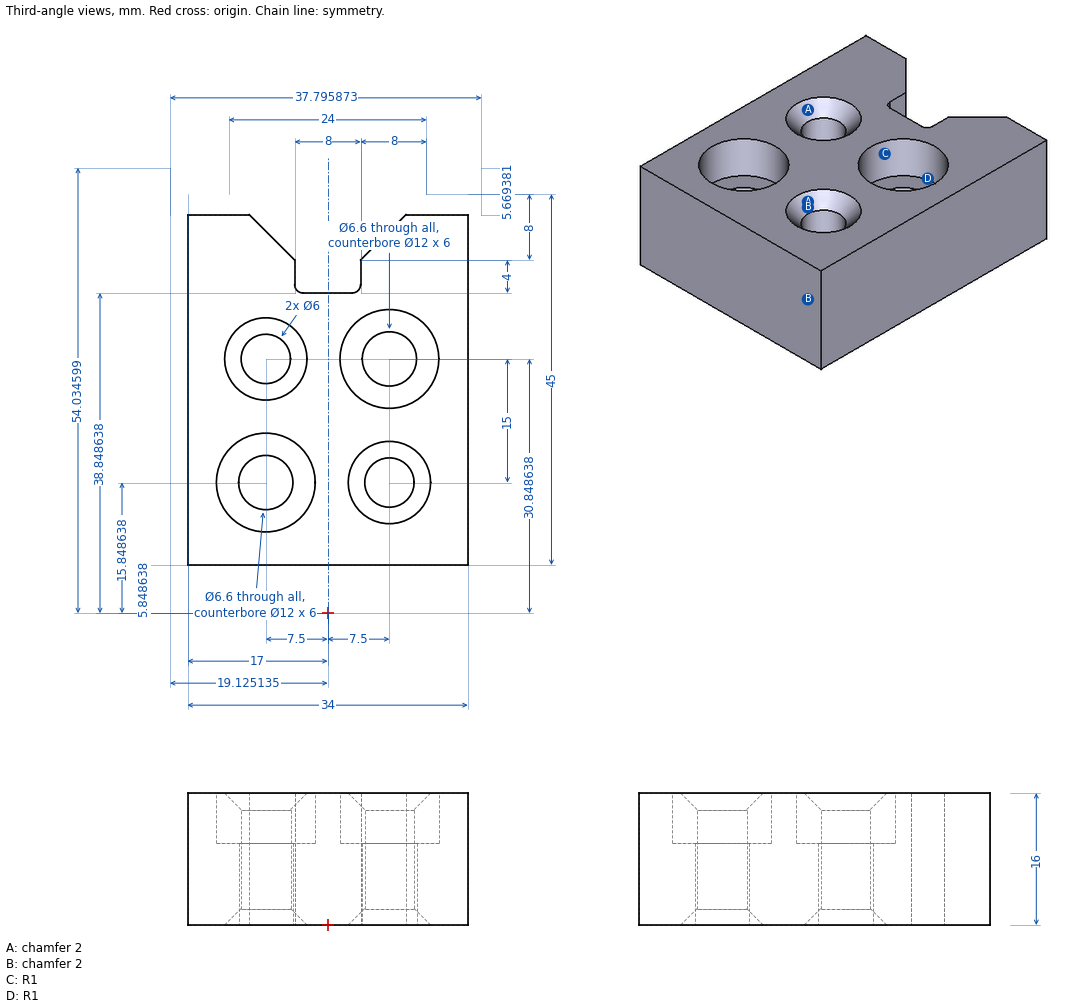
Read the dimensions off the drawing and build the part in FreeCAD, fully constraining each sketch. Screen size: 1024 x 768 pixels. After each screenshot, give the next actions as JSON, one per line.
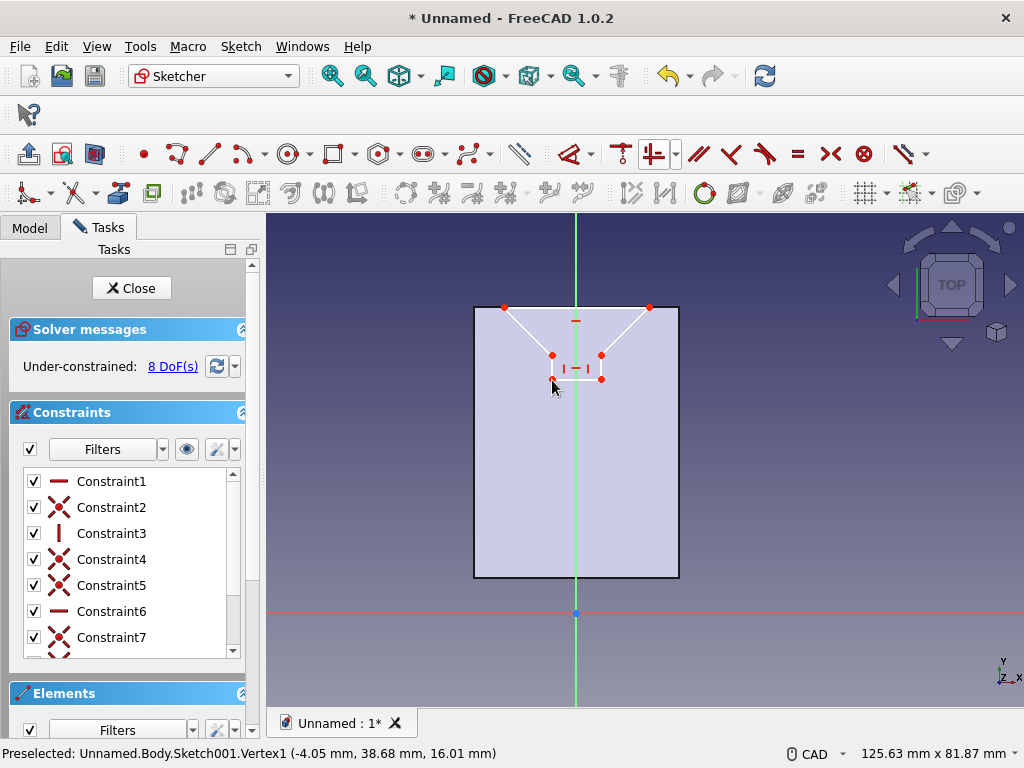
{"action": "left_click", "coordinate": [601, 356]}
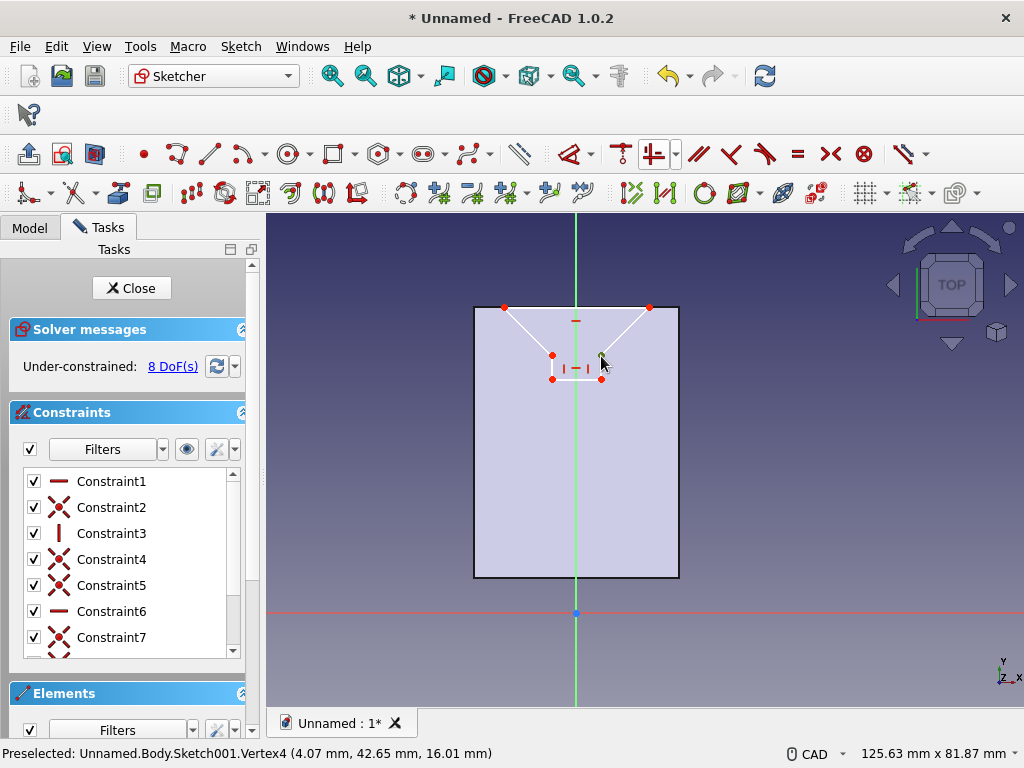
{"action": "left_click", "coordinate": [552, 356]}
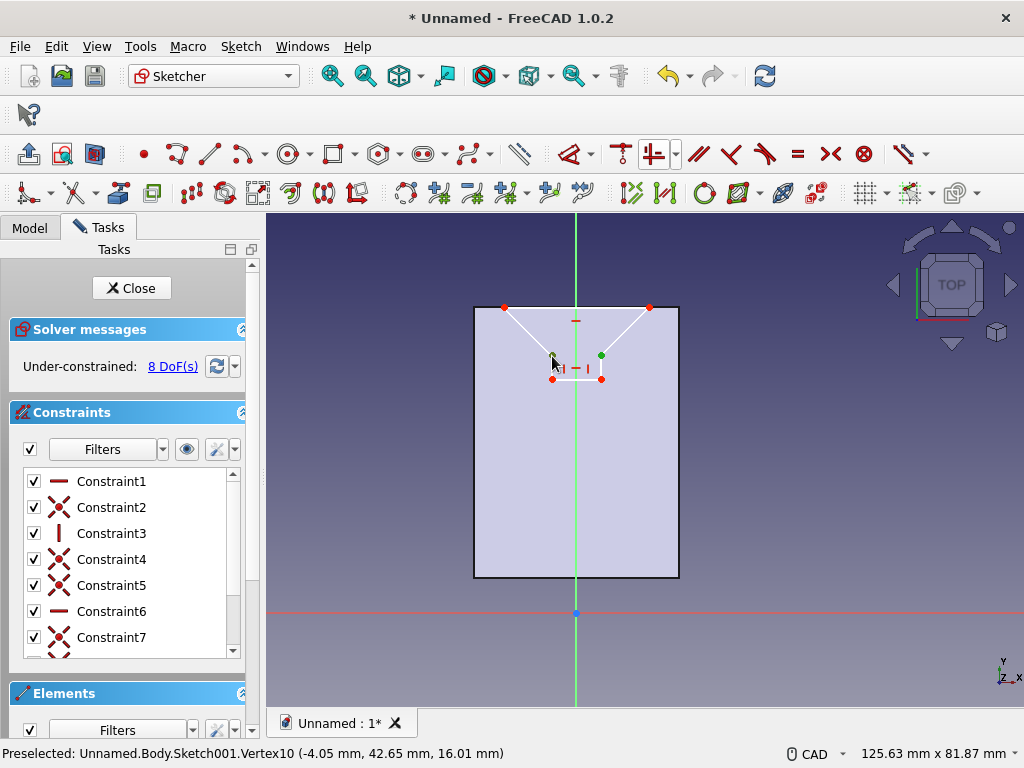
{"action": "left_click", "coordinate": [576, 648]}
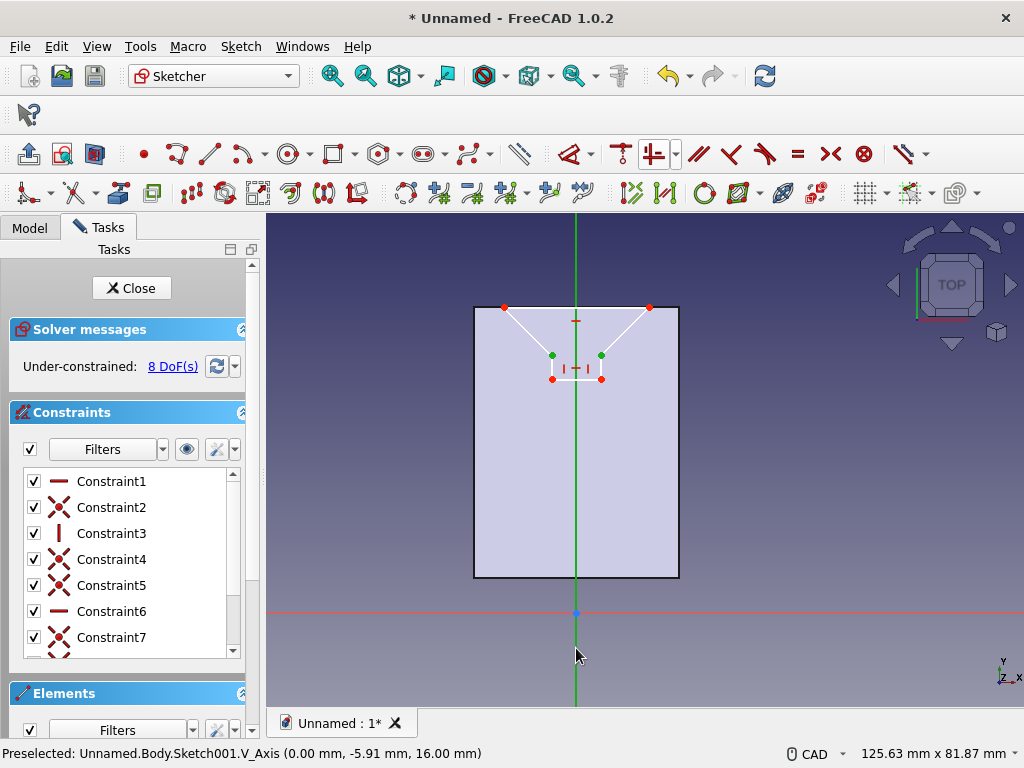
{"action": "key", "text": "s"}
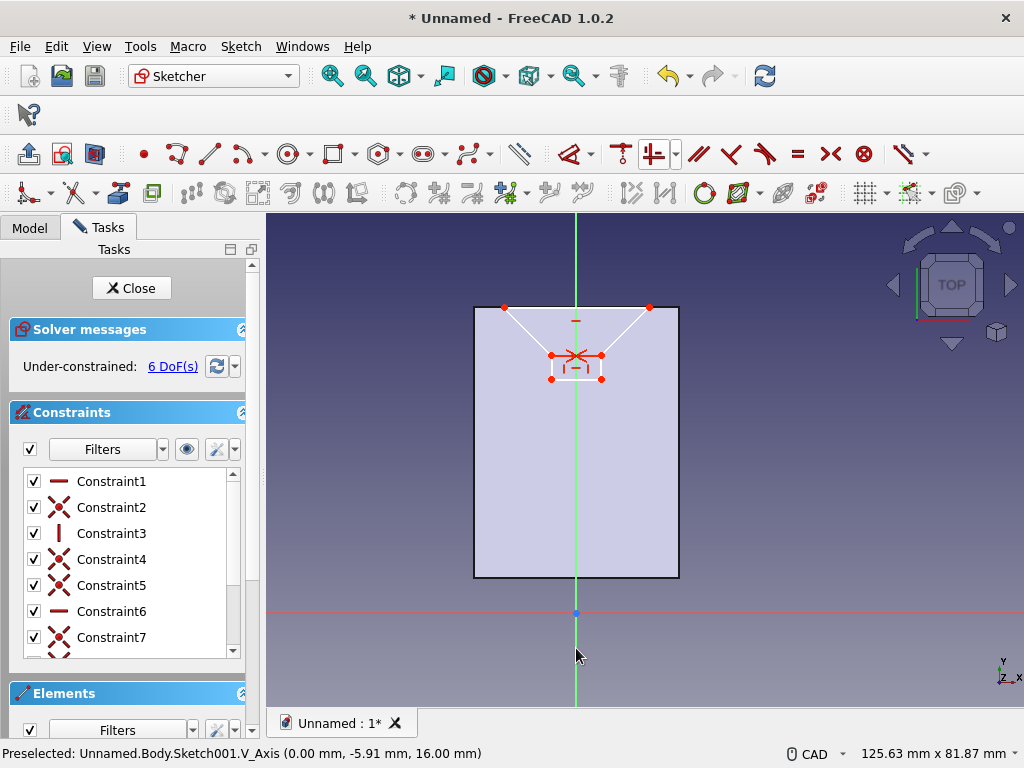
{"action": "left_click", "coordinate": [568, 154]}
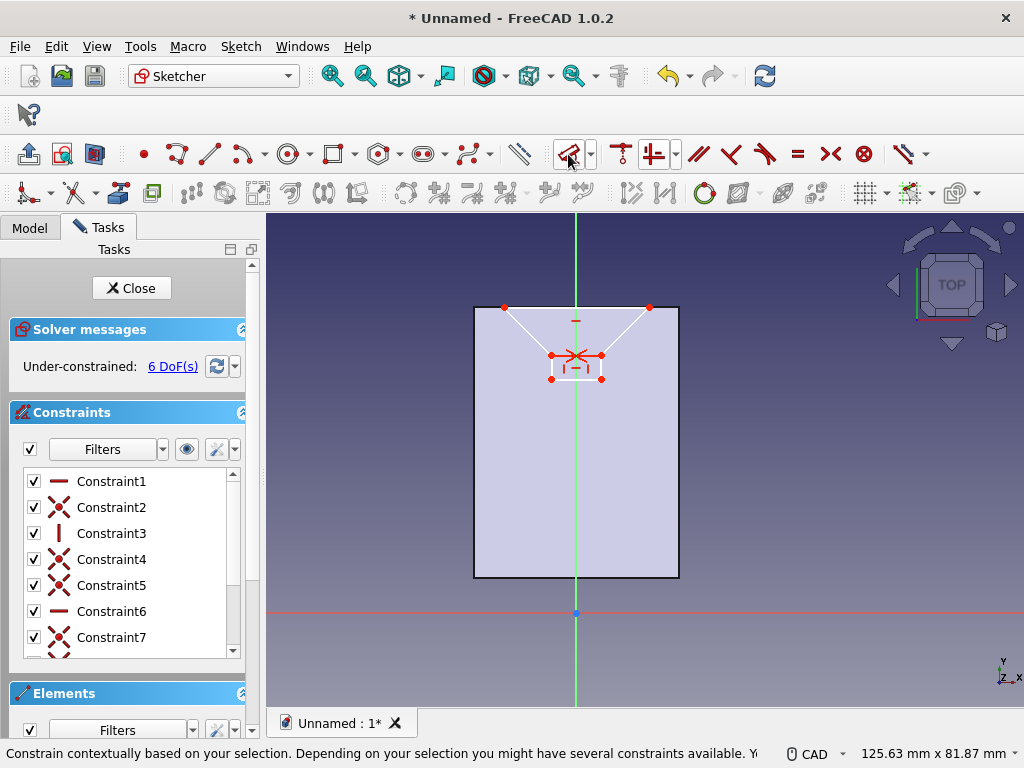
{"action": "scroll", "coordinate": [567, 380], "scroll_direction": "up", "scroll_amount": 2}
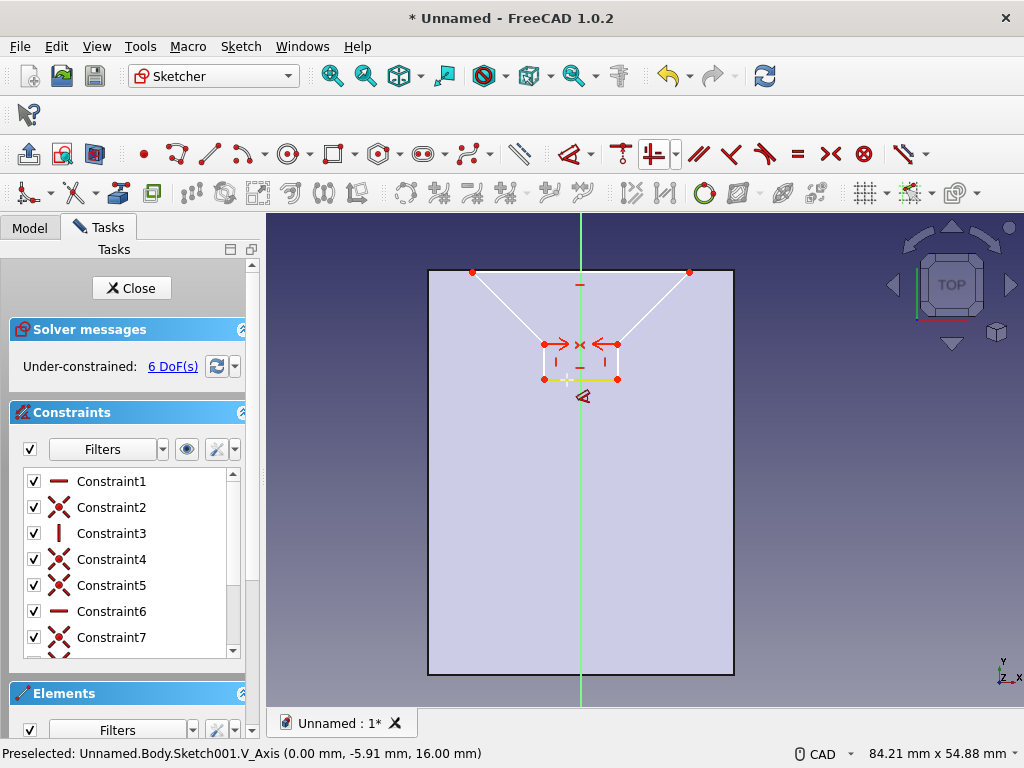
{"action": "left_click", "coordinate": [566, 380]}
{"action": "left_click", "coordinate": [564, 346]}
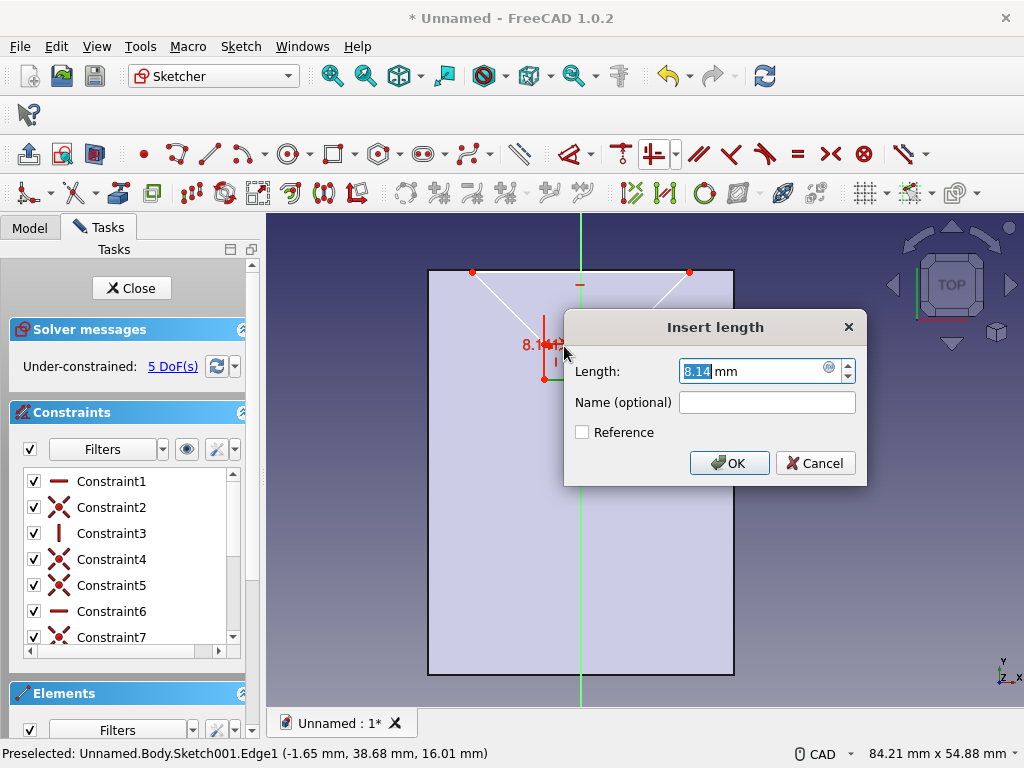
{"action": "type", "text": "8"}
{"action": "key", "text": "Return"}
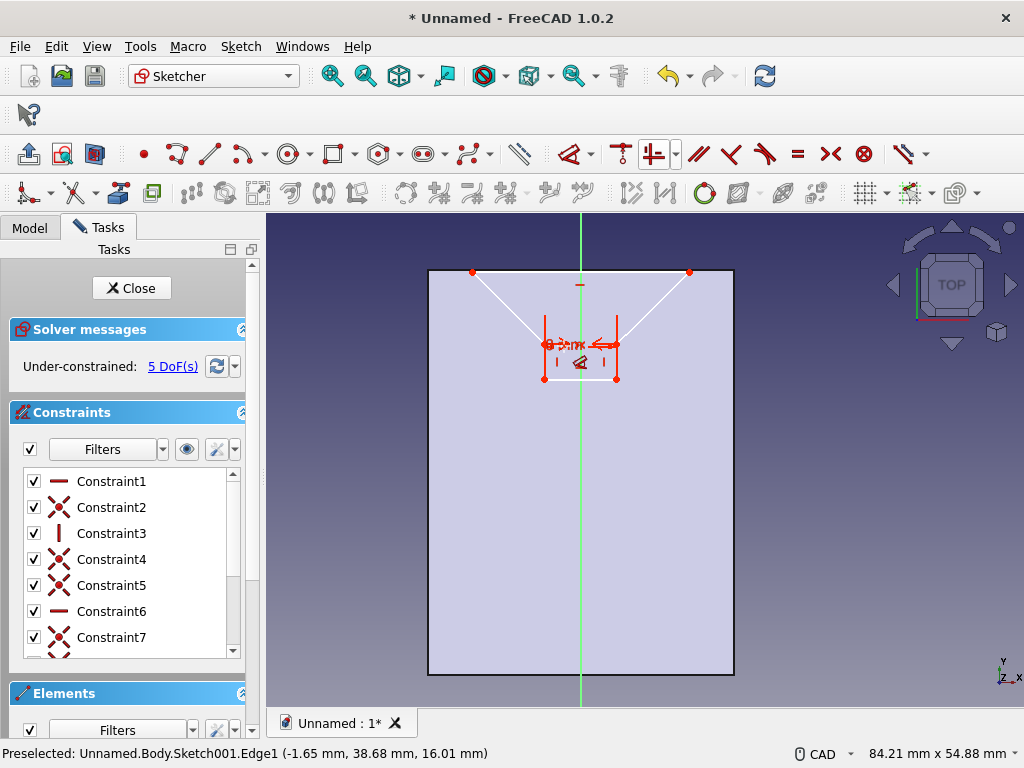
{"action": "scroll", "coordinate": [617, 369], "scroll_direction": "up", "scroll_amount": 2}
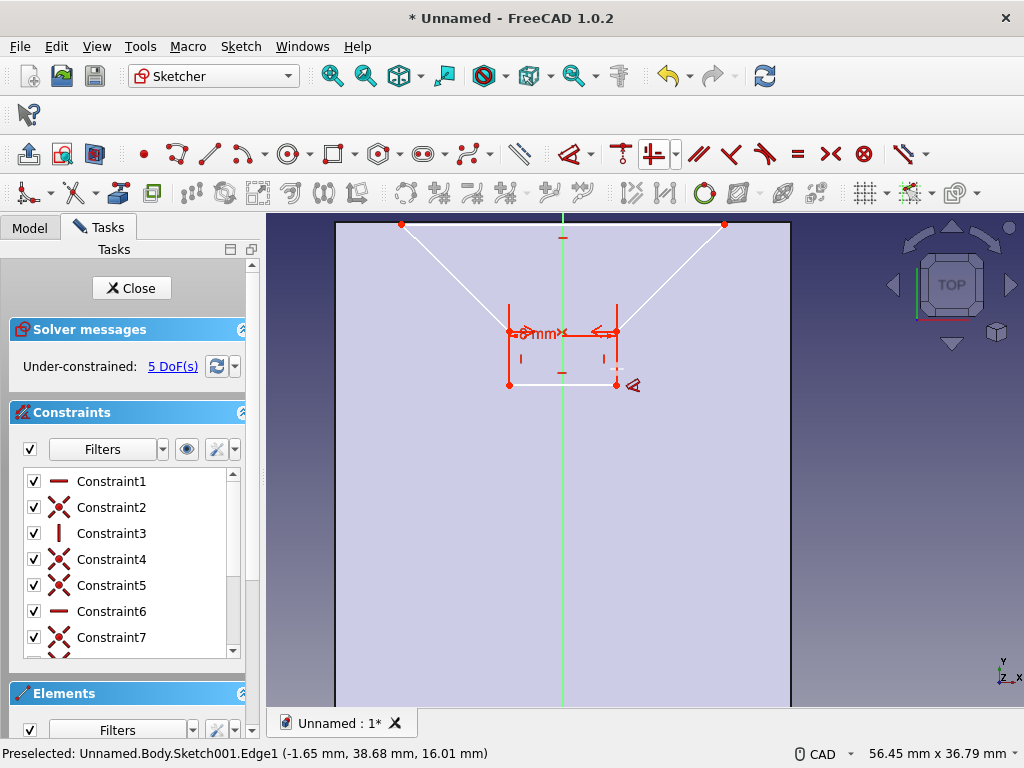
{"action": "left_click", "coordinate": [617, 369]}
{"action": "left_click", "coordinate": [651, 358]}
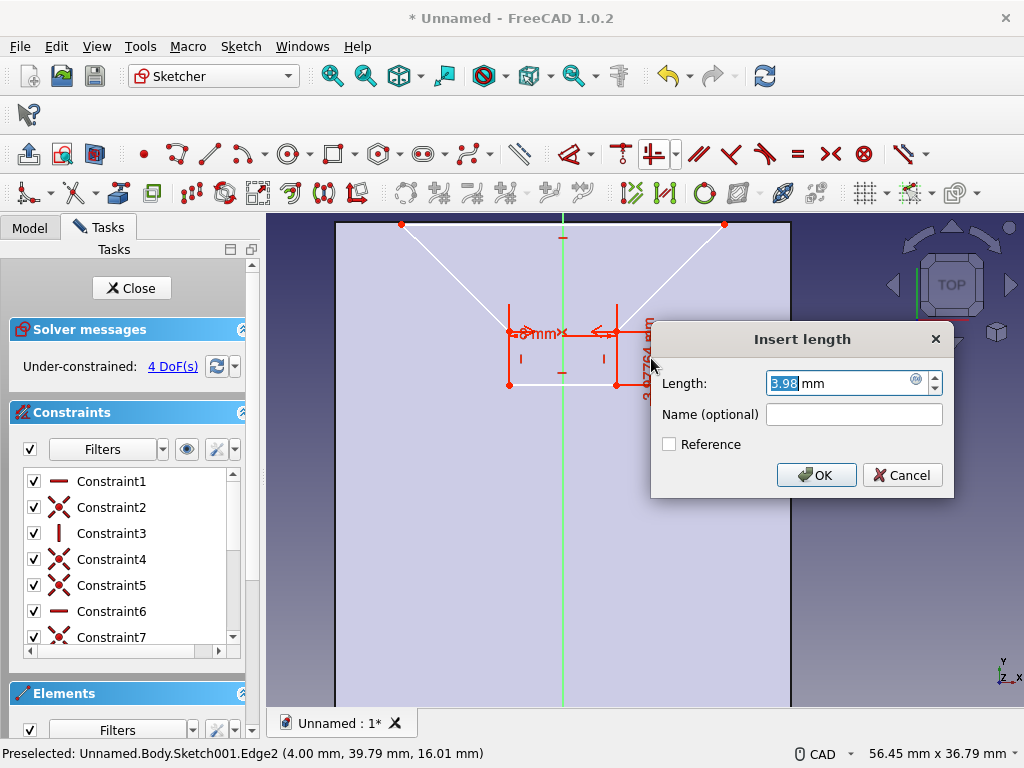
{"action": "type", "text": "4"}
{"action": "key", "text": "Return"}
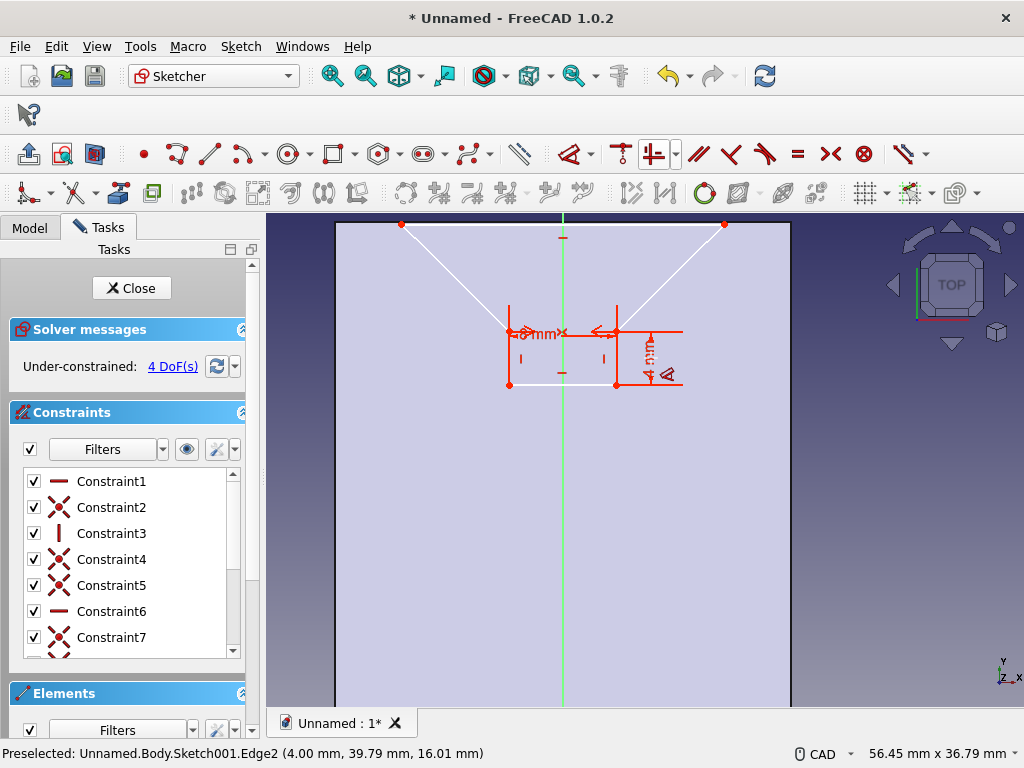
{"action": "scroll", "coordinate": [588, 376], "scroll_direction": "down", "scroll_amount": 4}